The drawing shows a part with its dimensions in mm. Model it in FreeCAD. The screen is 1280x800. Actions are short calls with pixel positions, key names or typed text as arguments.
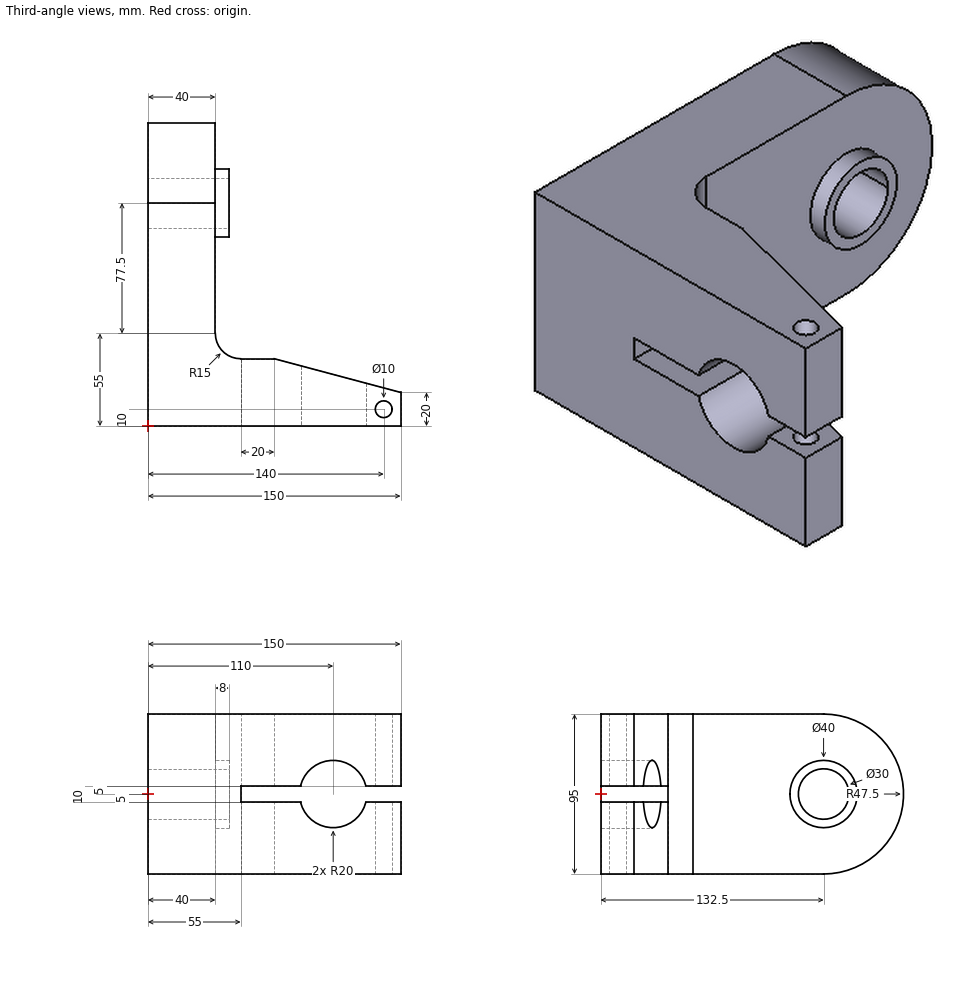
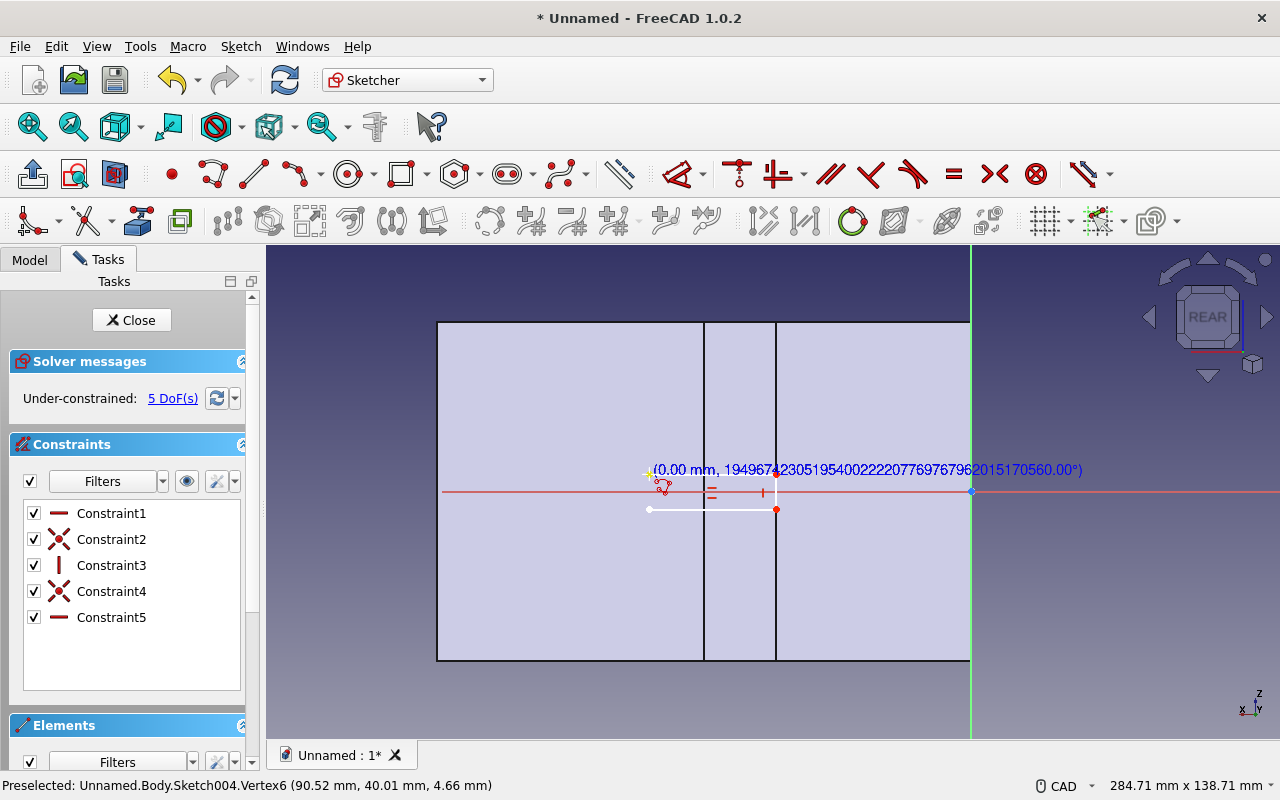
click(511, 474)
click(437, 474)
click(437, 509)
click(511, 509)
right_click(511, 509)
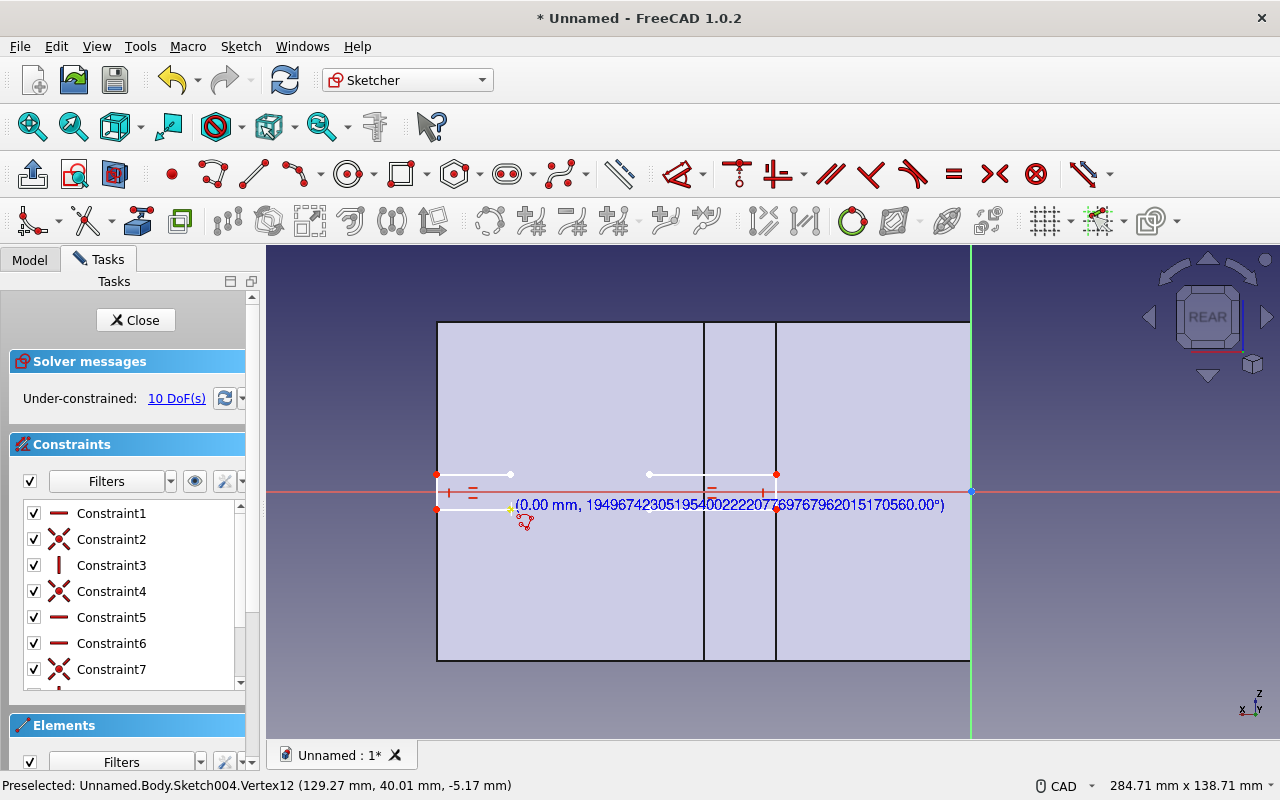
click(294, 174)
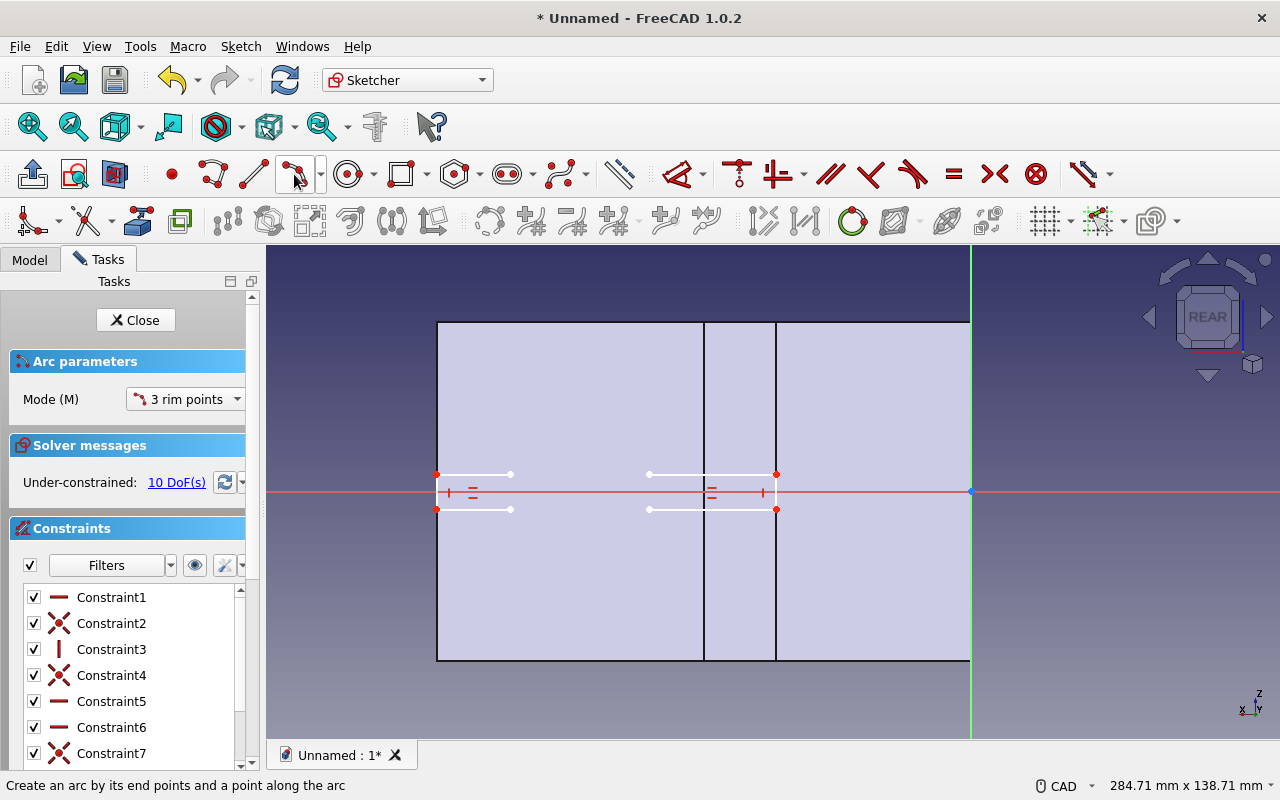
click(649, 475)
click(511, 475)
click(580, 420)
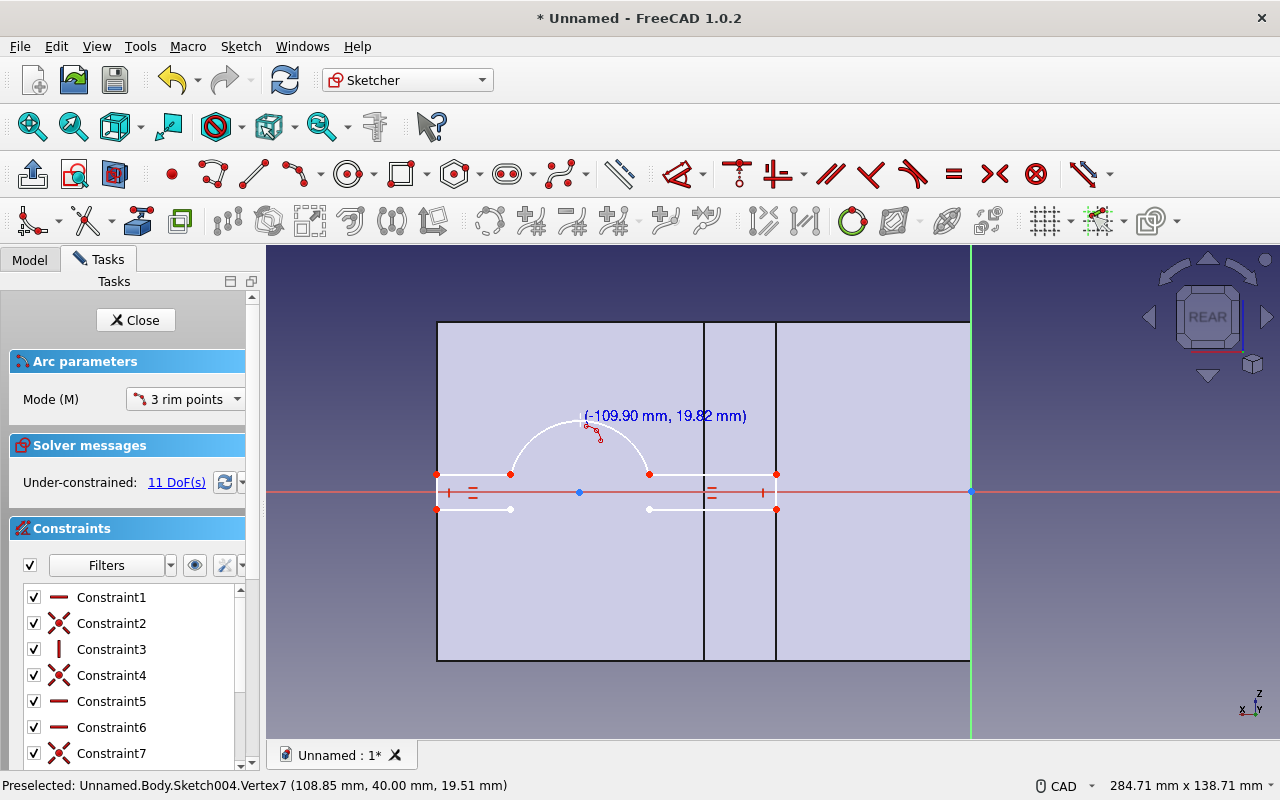
click(511, 510)
click(649, 510)
click(580, 563)
key(Escape)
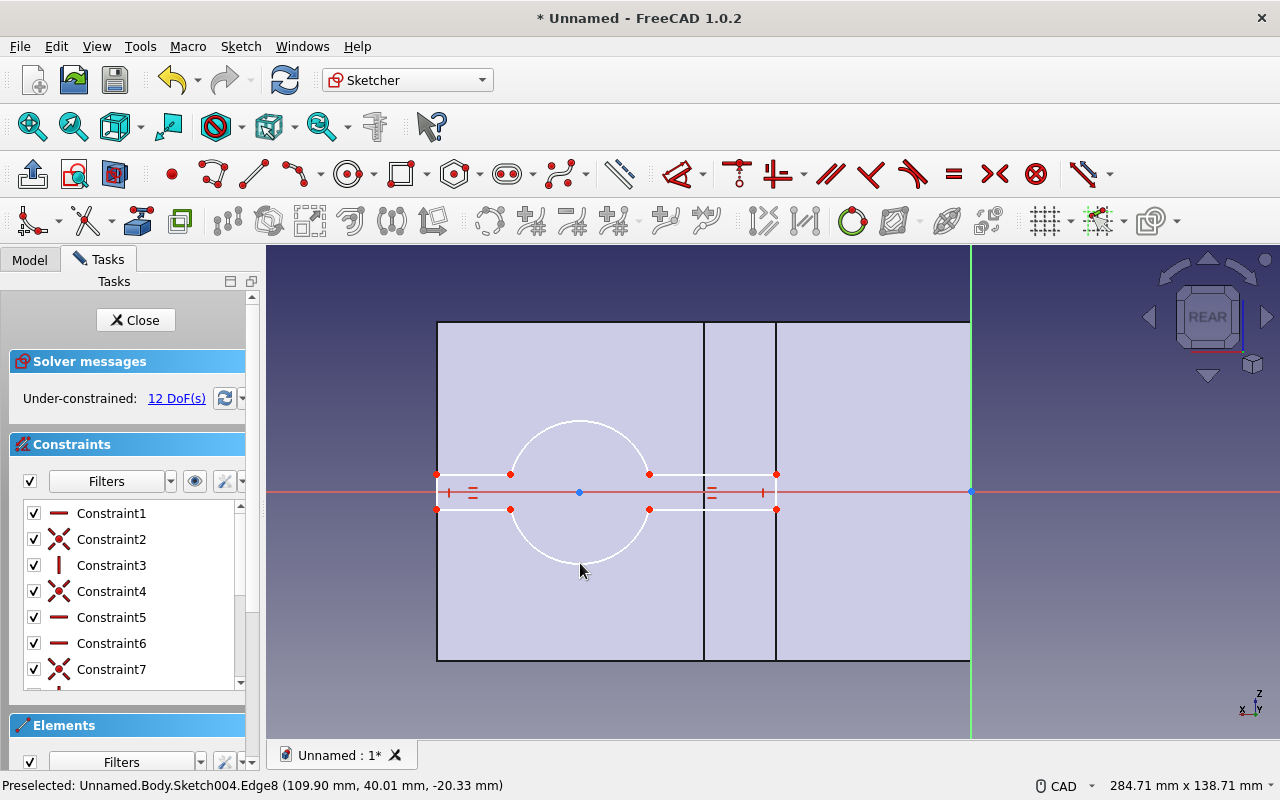
click(616, 431)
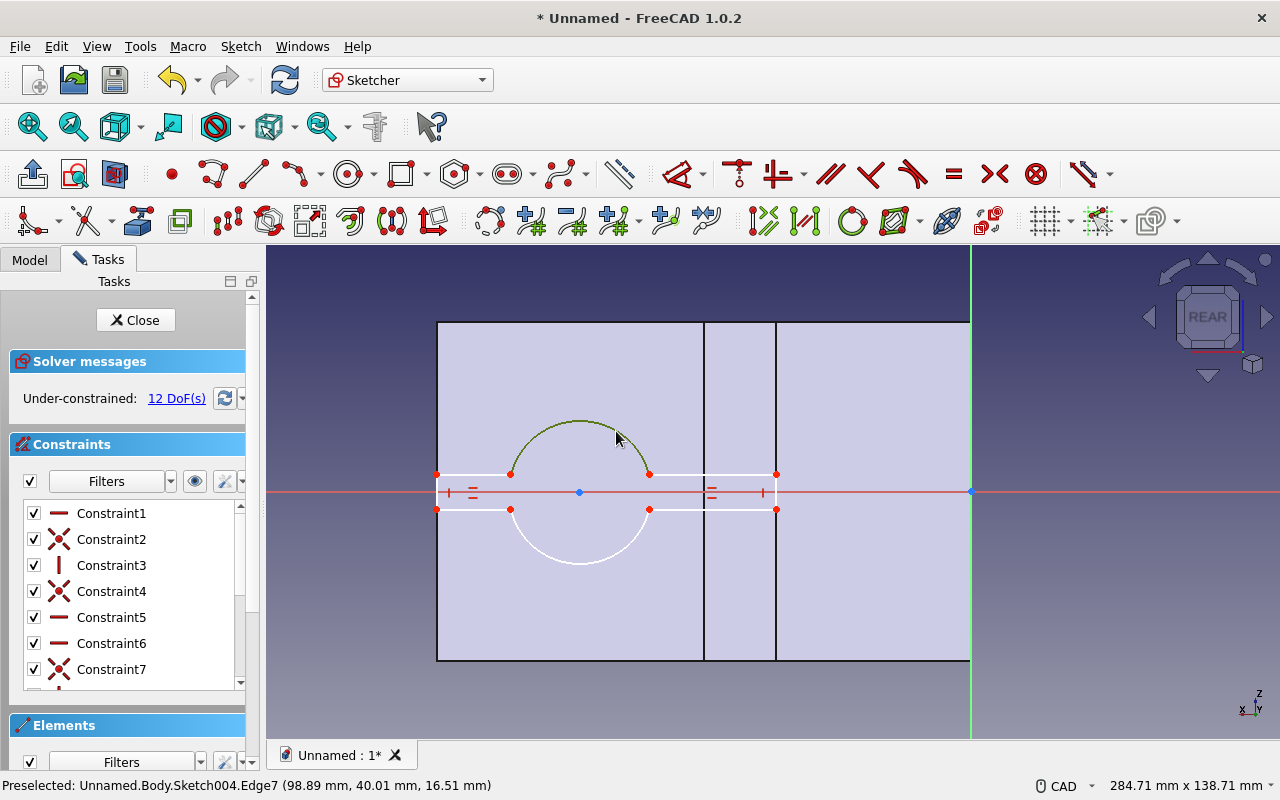
click(544, 554)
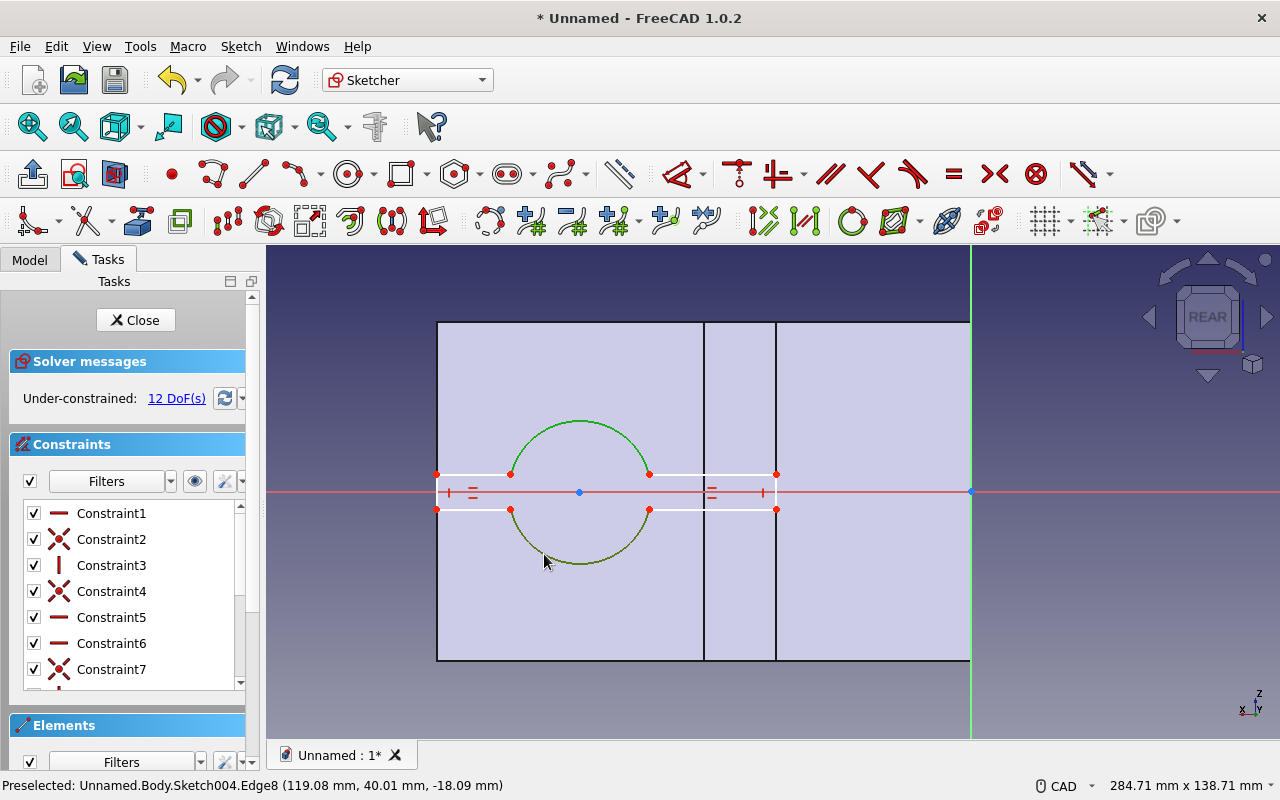
click(737, 174)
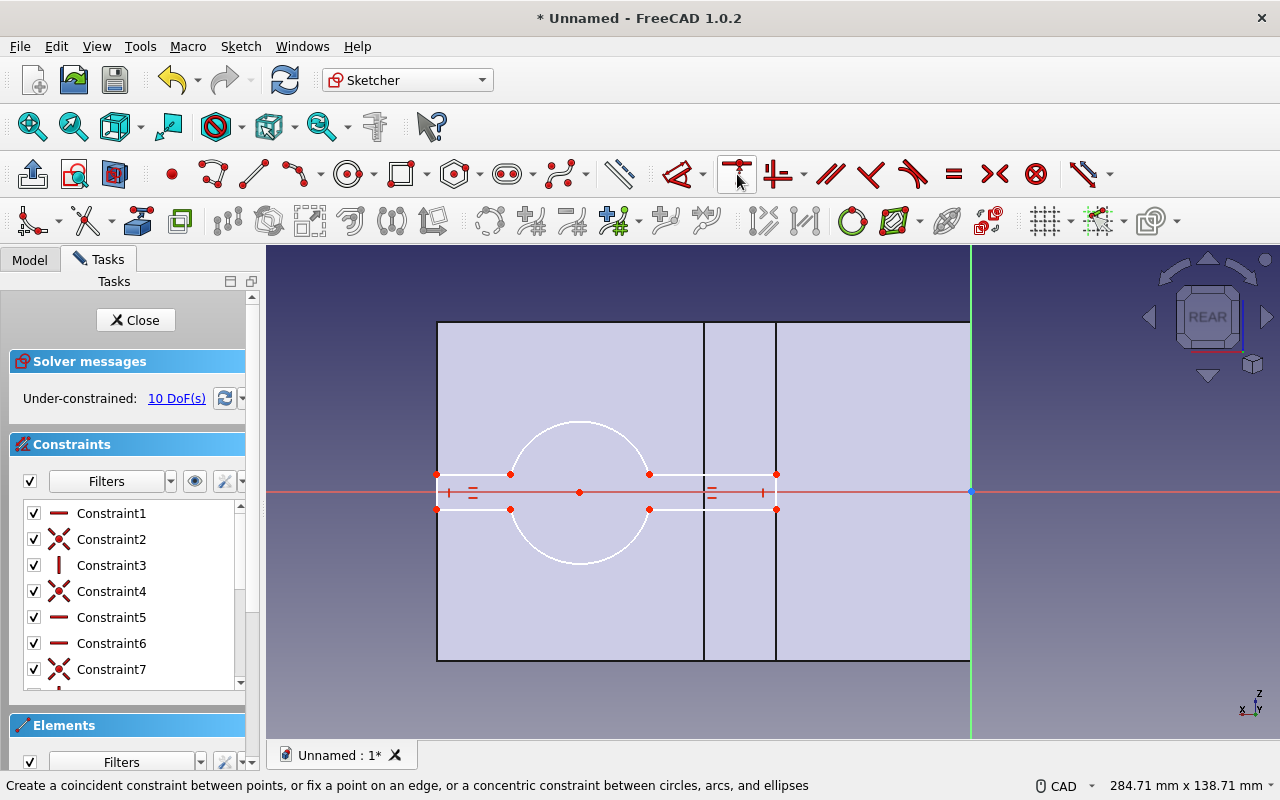
click(616, 431)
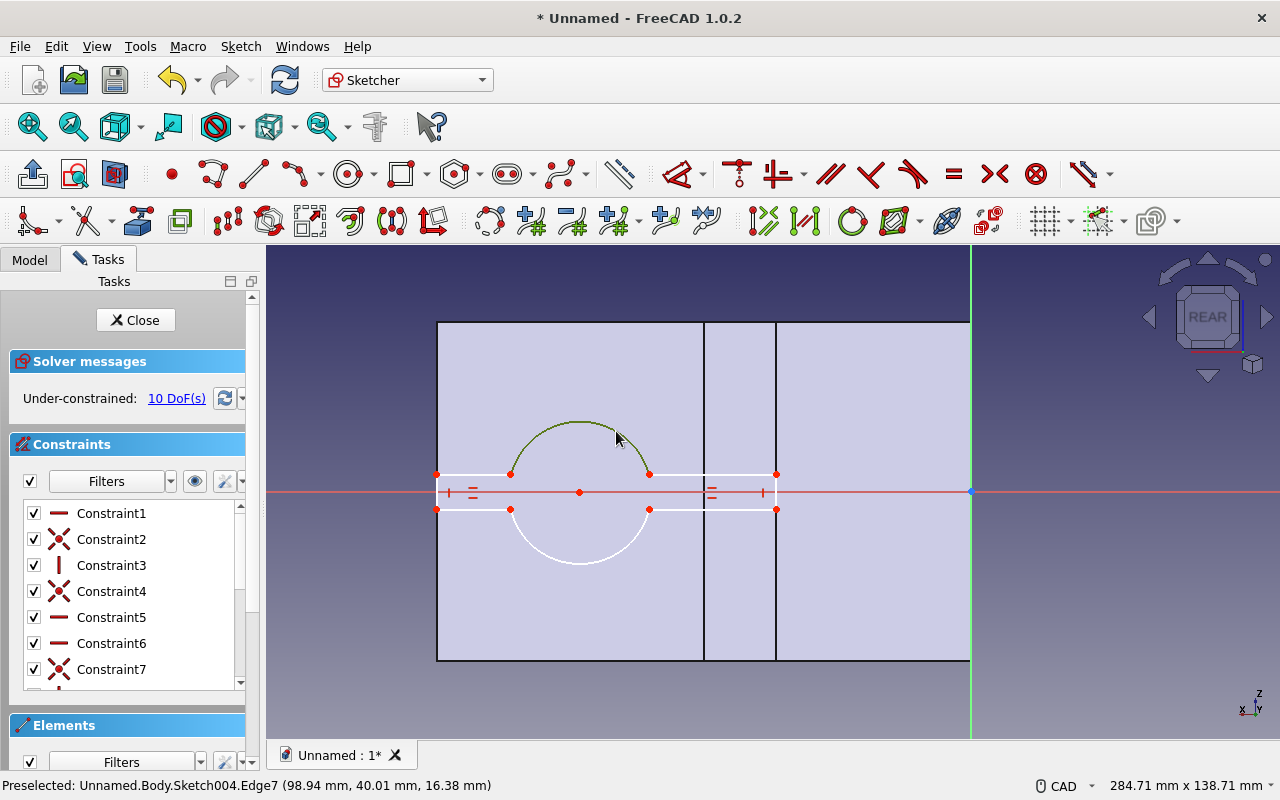
click(544, 554)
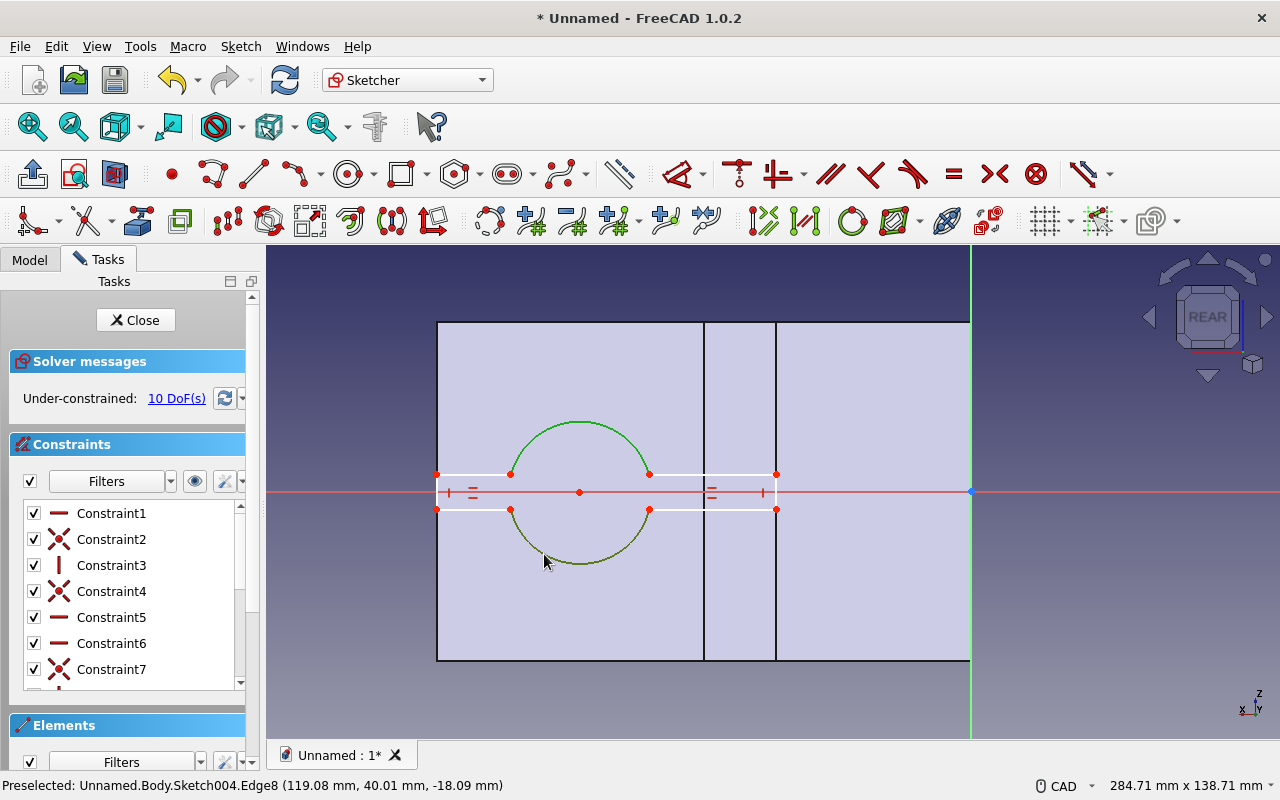
click(954, 174)